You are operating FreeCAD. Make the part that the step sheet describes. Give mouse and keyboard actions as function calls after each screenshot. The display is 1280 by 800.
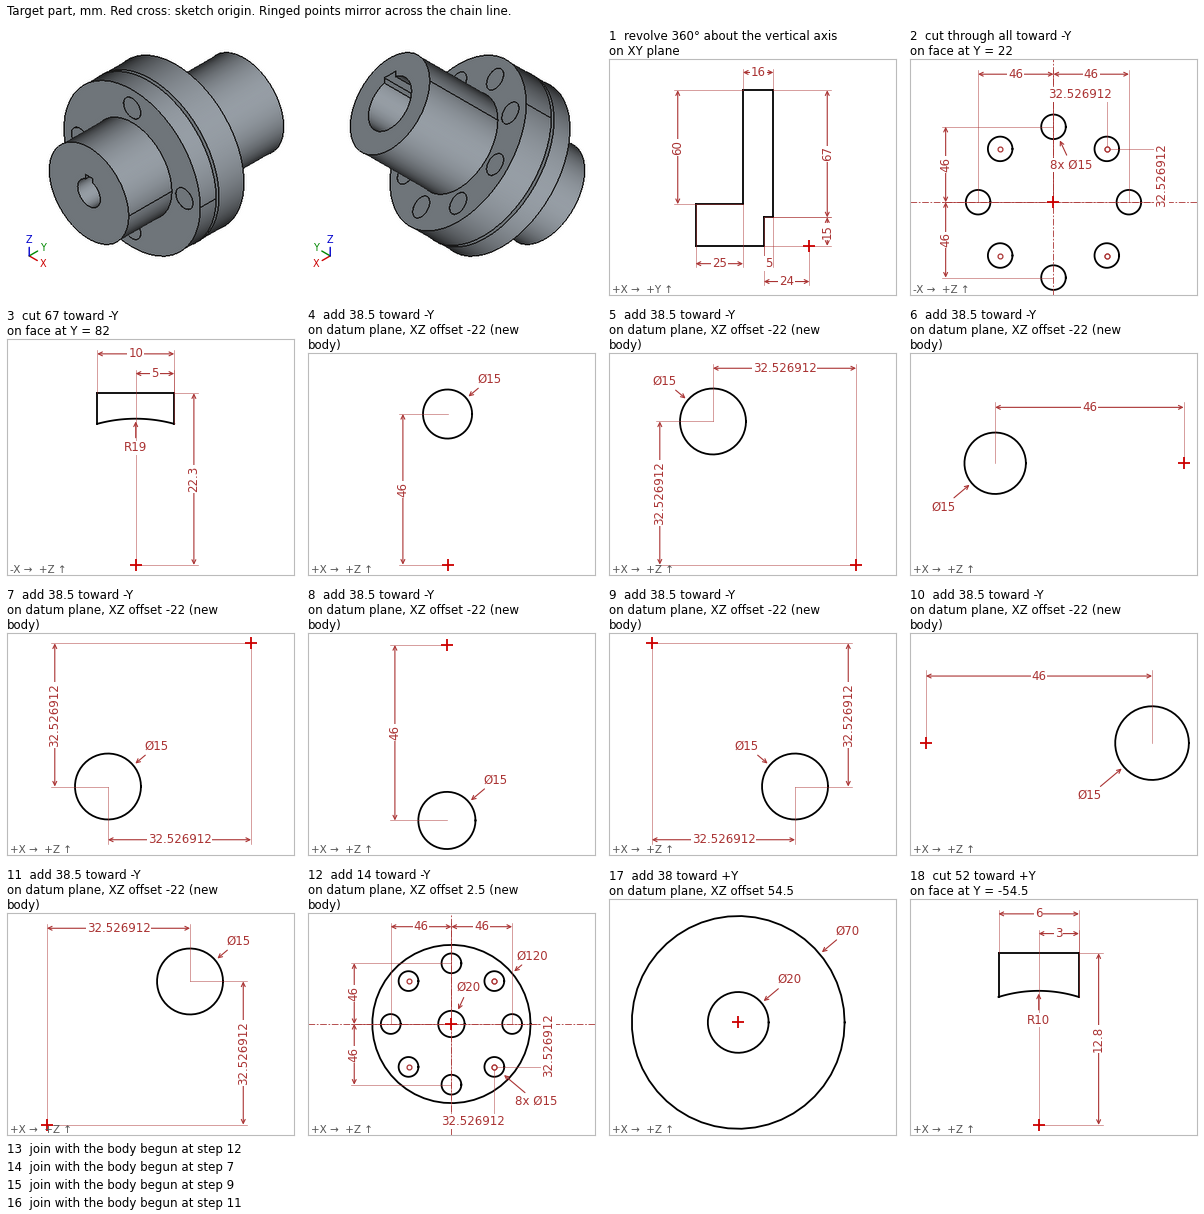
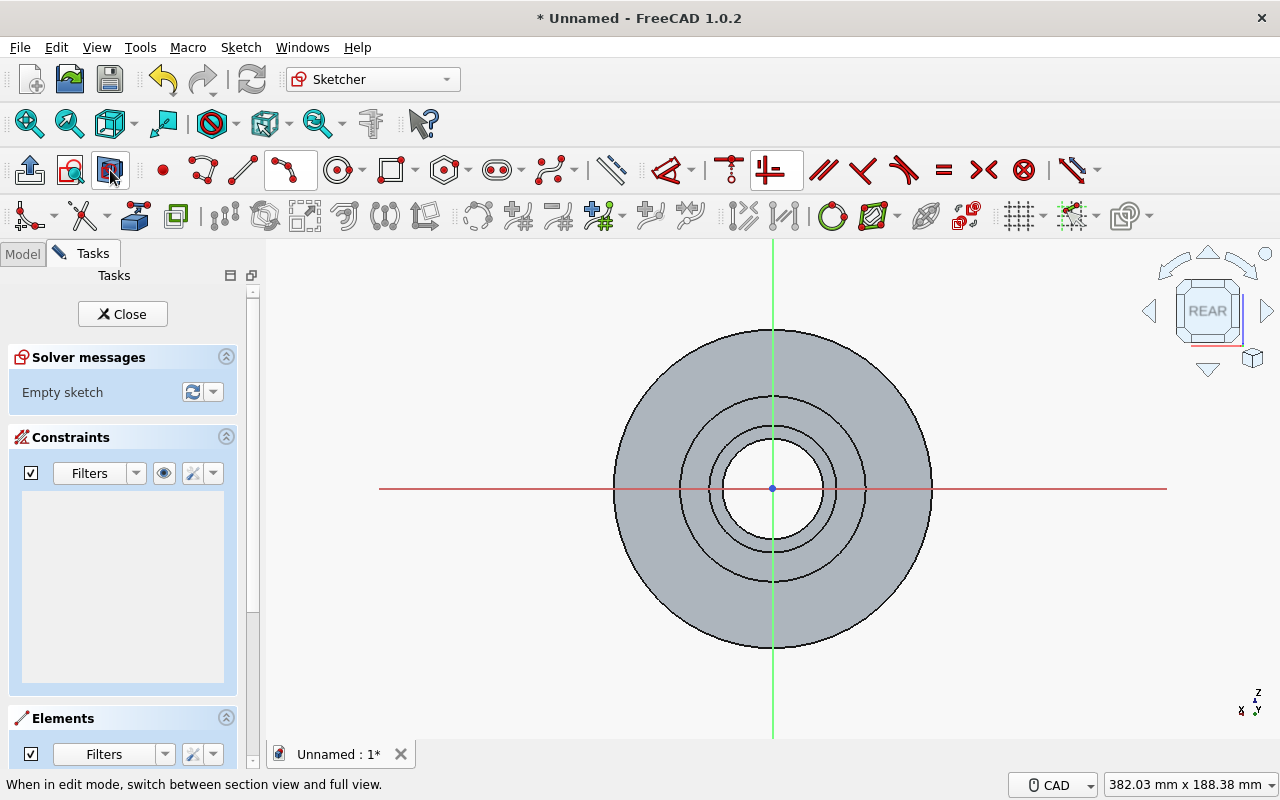
click(338, 170)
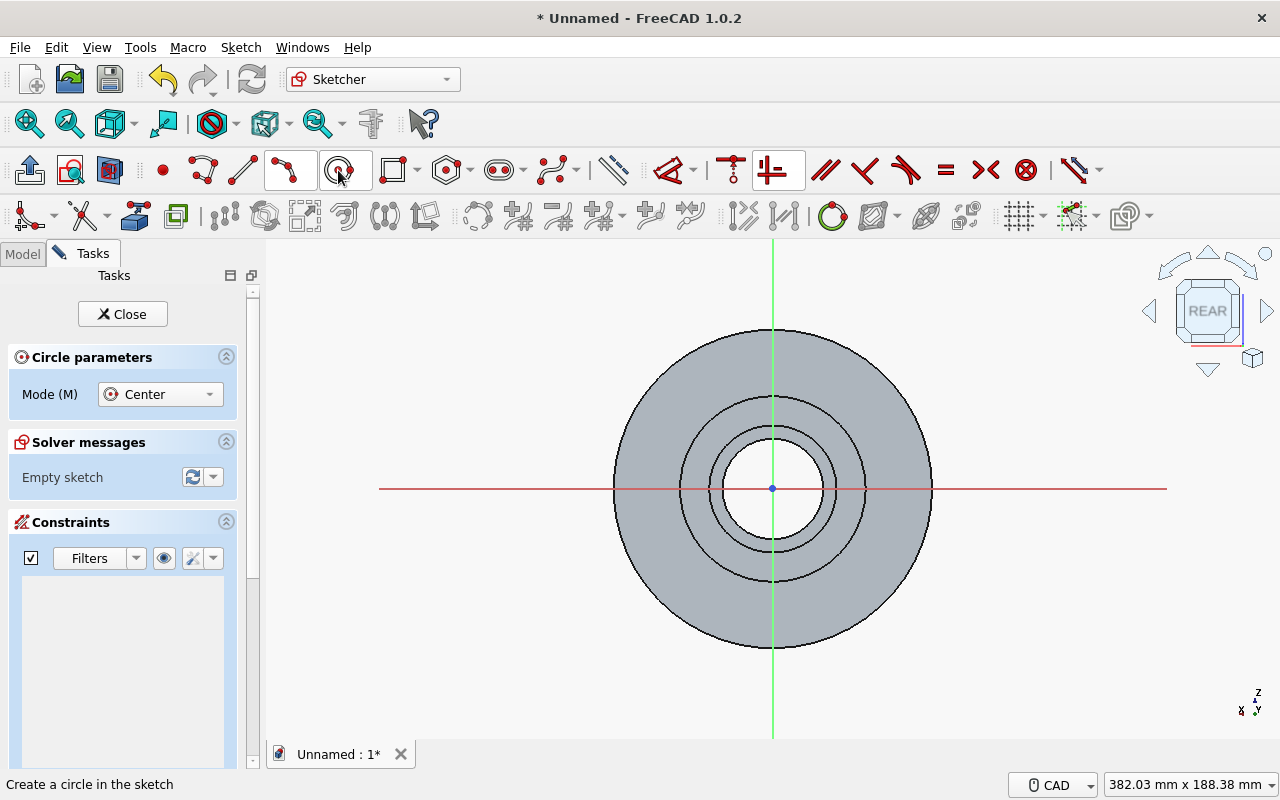
click(773, 367)
click(787, 353)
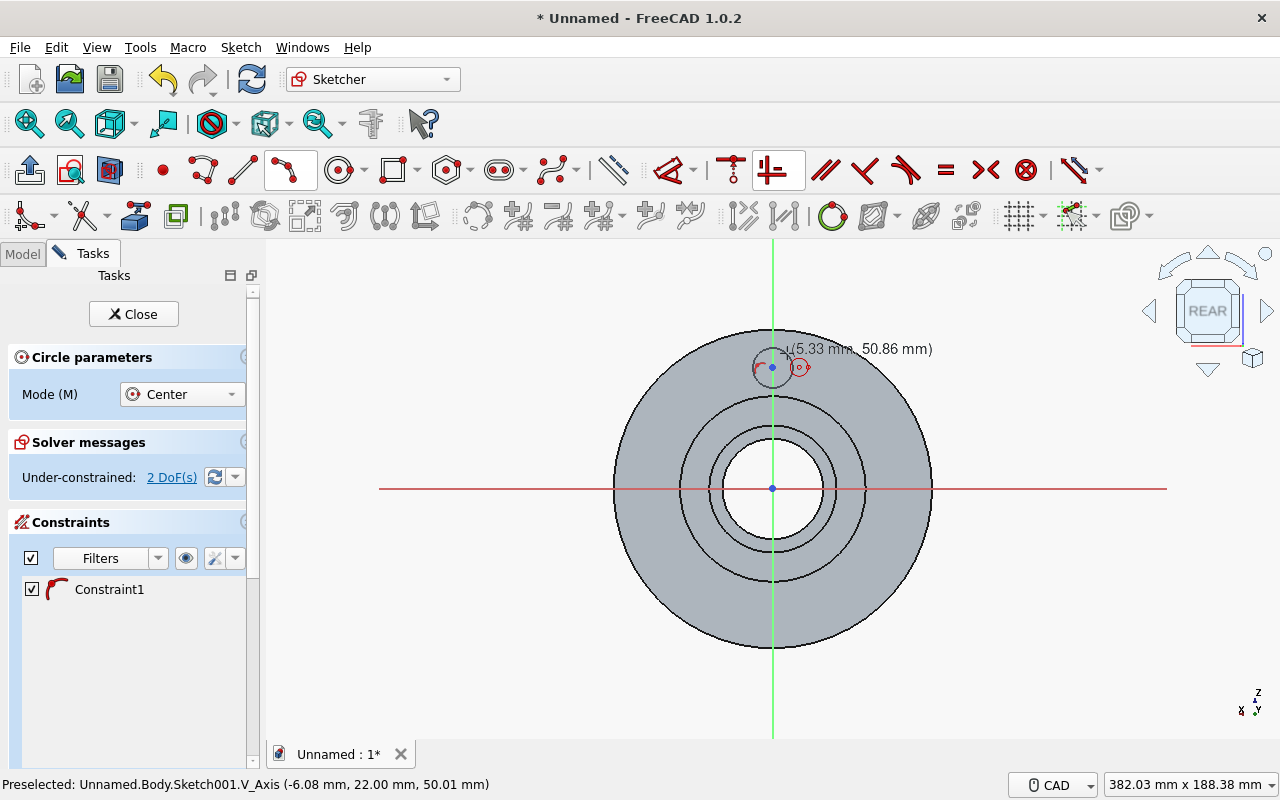
click(859, 403)
click(873, 389)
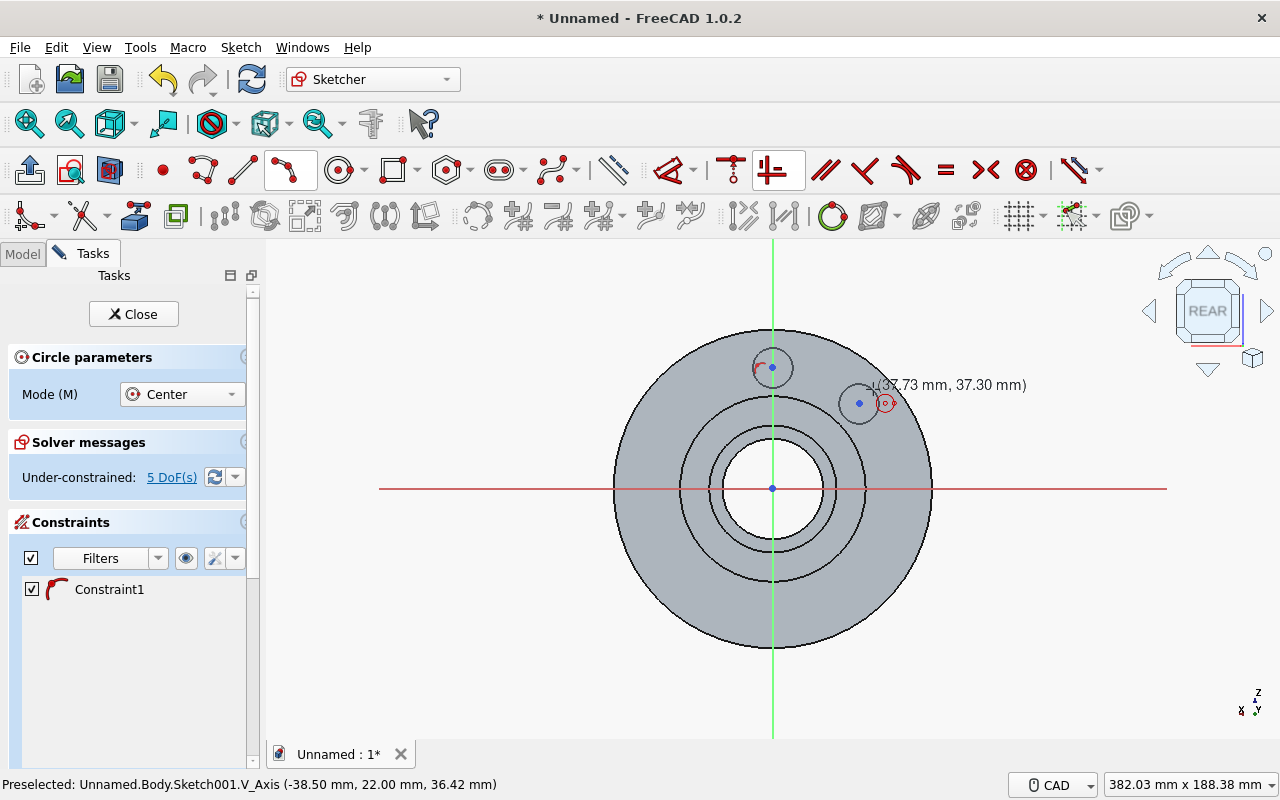
click(895, 489)
click(909, 475)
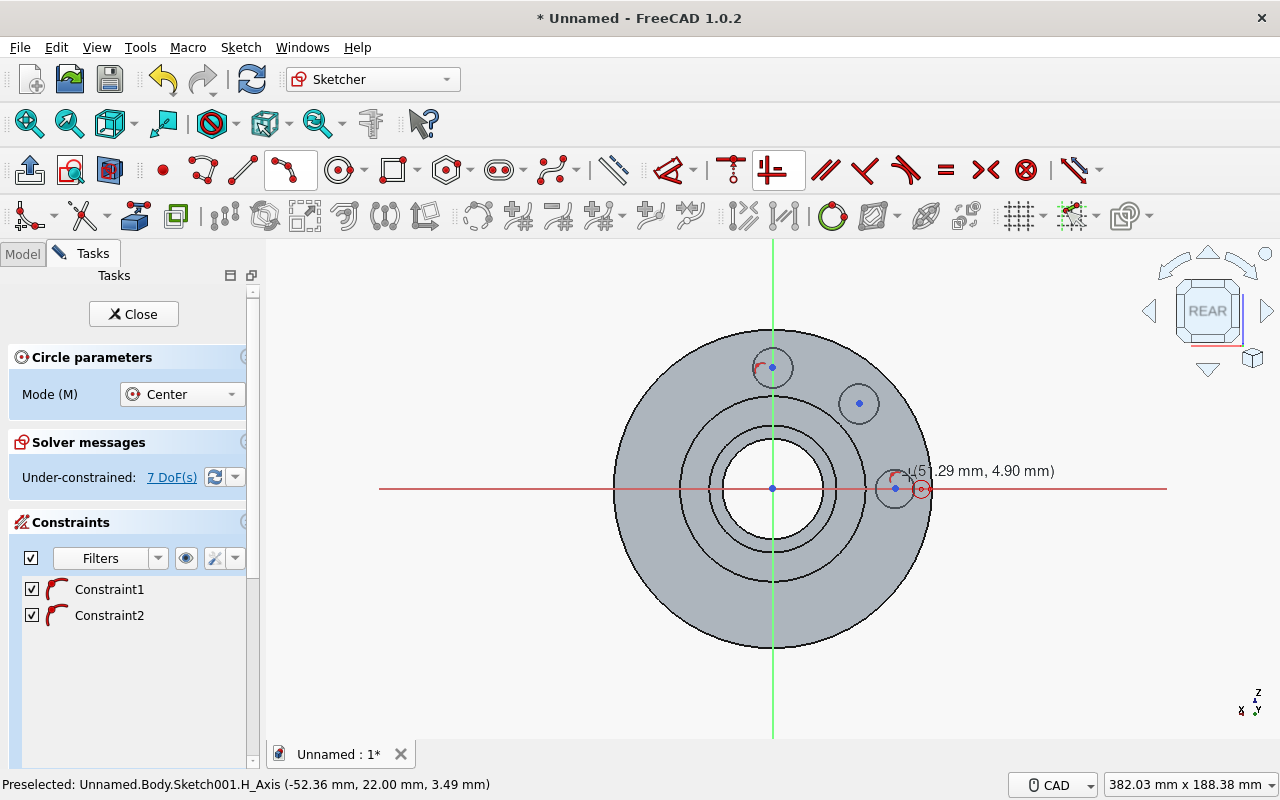
click(859, 575)
click(873, 561)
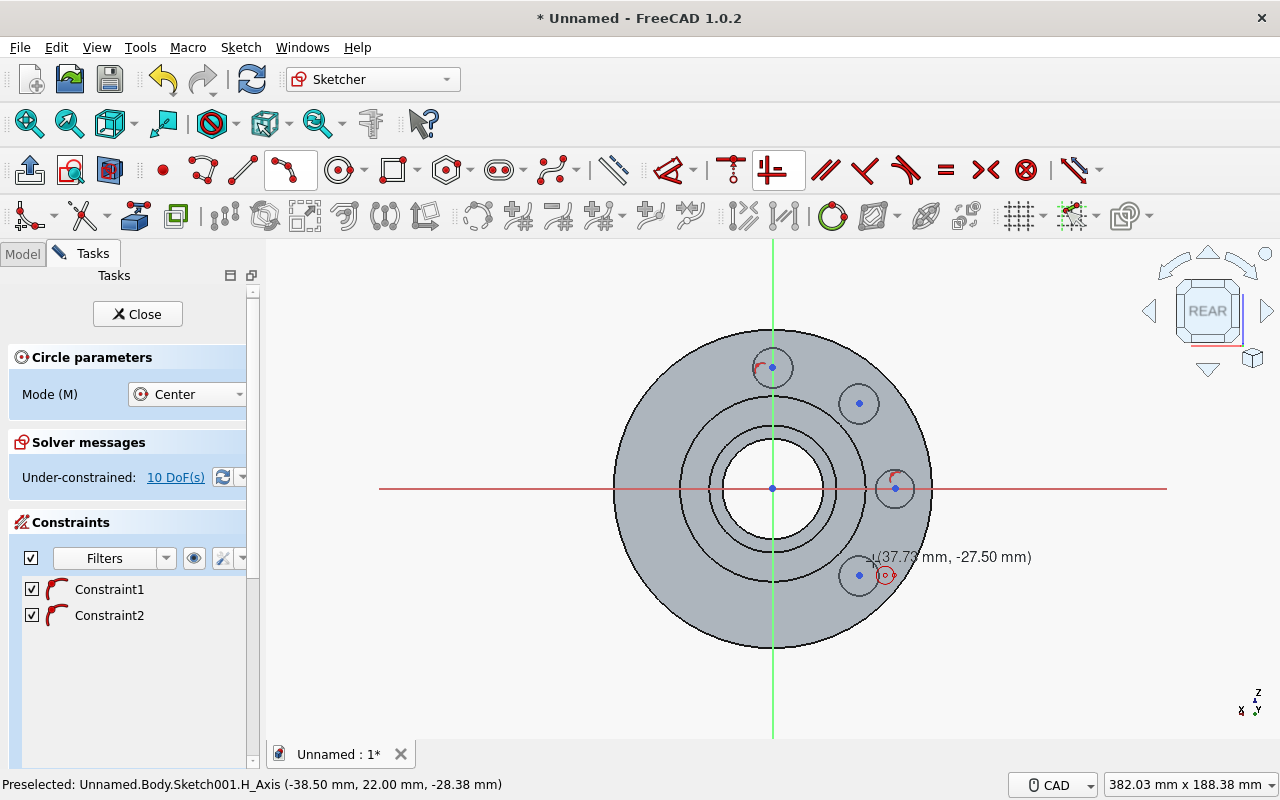
click(773, 611)
click(787, 597)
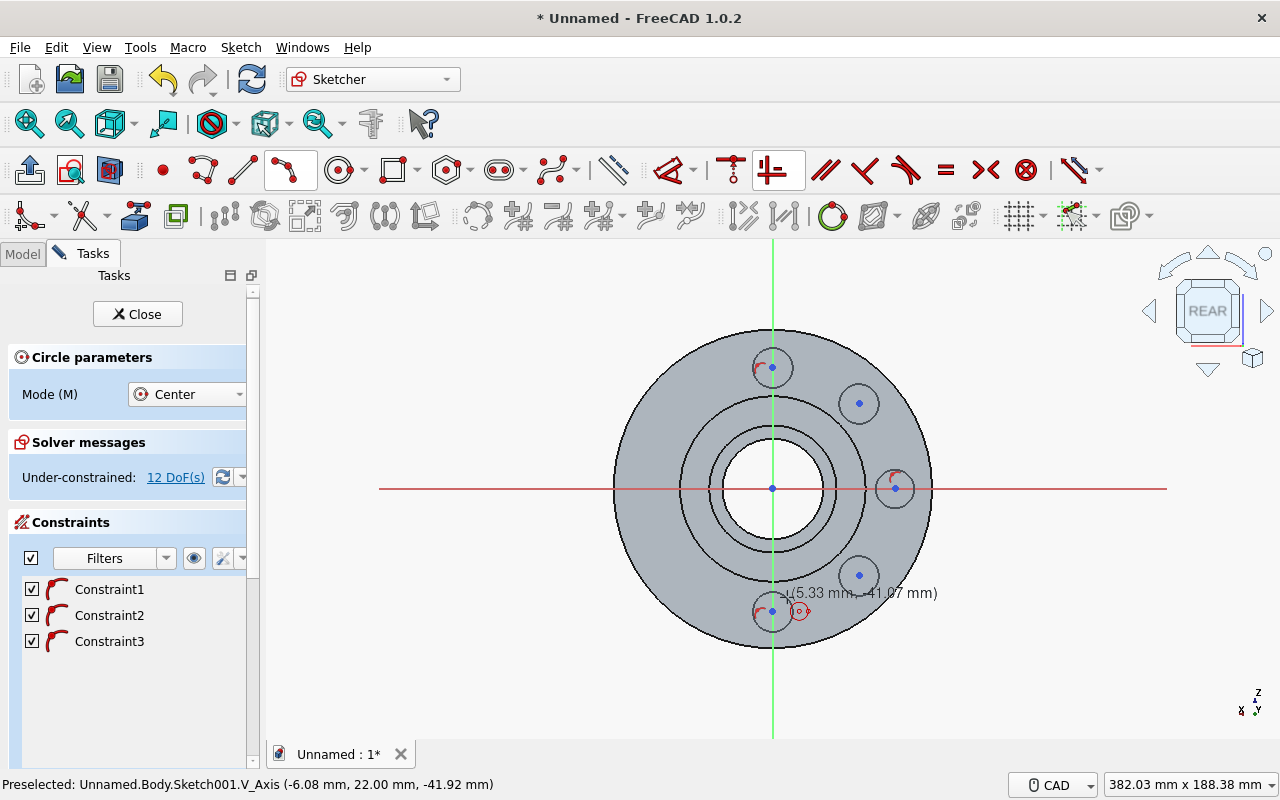
click(687, 575)
click(701, 561)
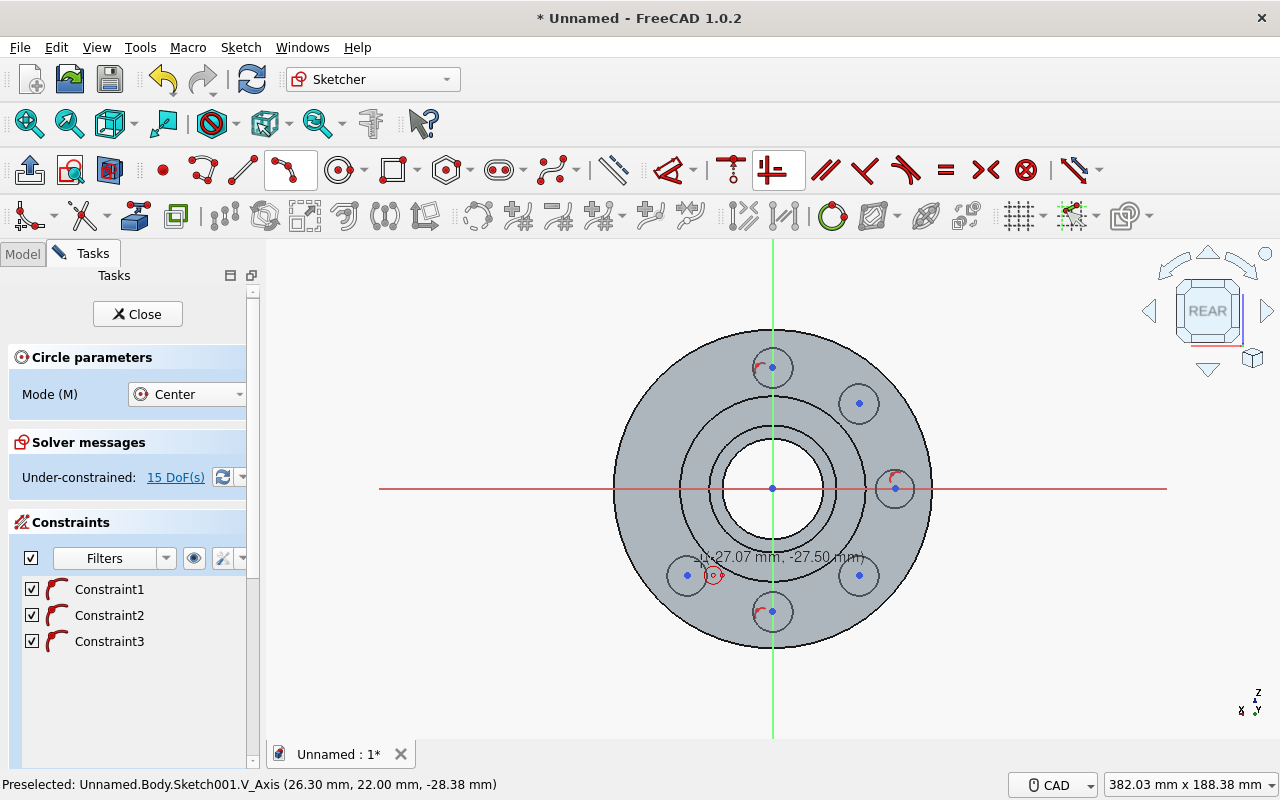
click(651, 489)
click(665, 475)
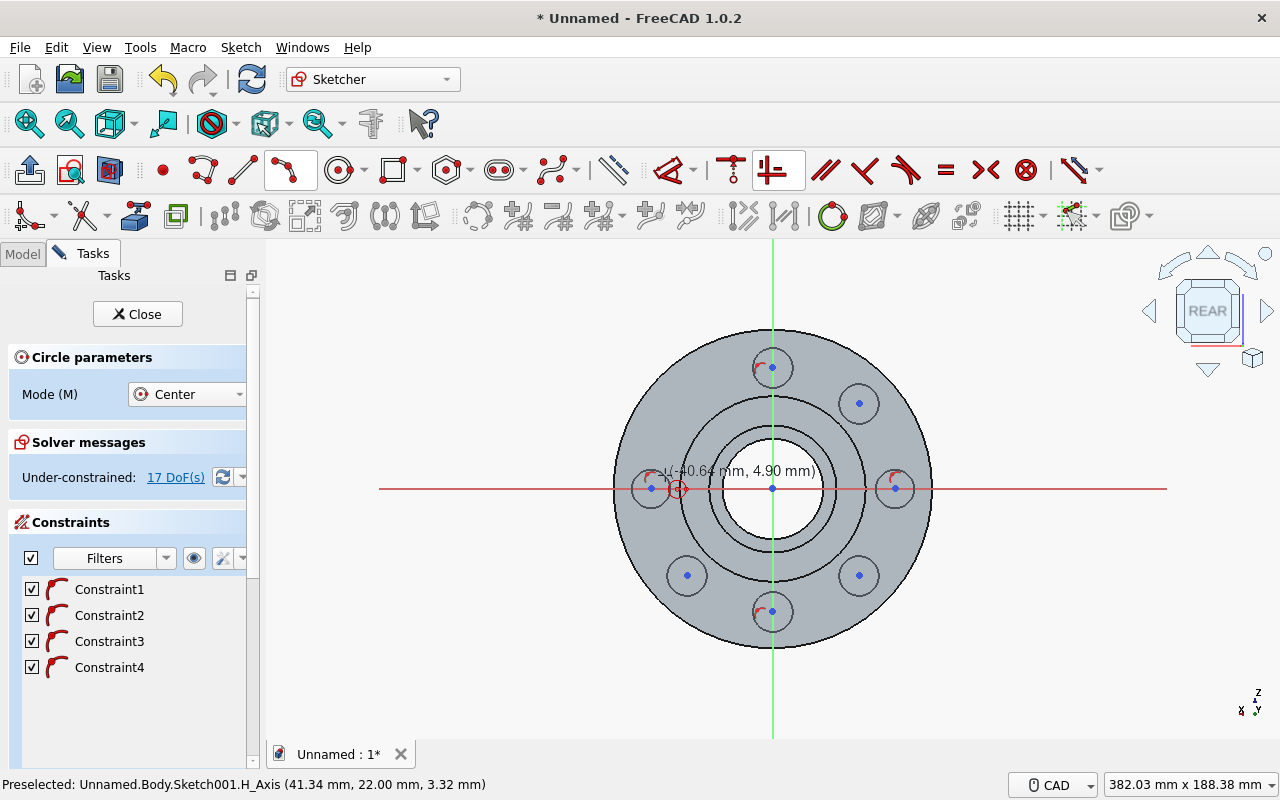
click(687, 403)
click(701, 389)
key(Escape)